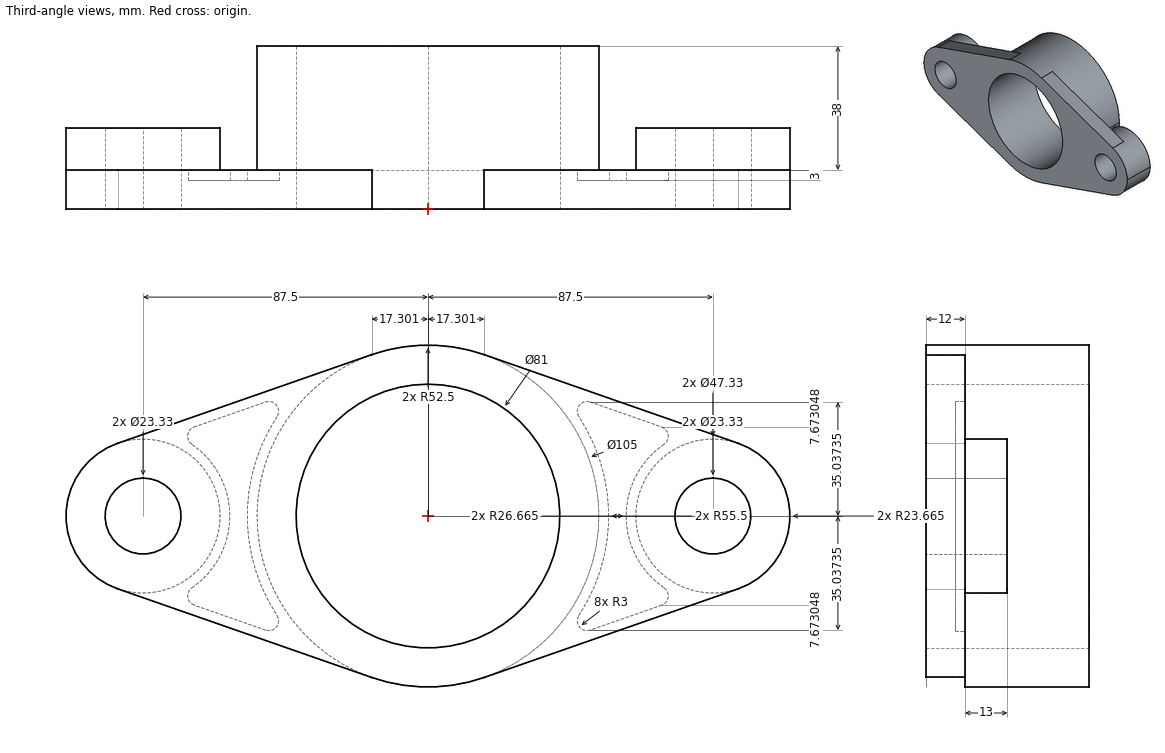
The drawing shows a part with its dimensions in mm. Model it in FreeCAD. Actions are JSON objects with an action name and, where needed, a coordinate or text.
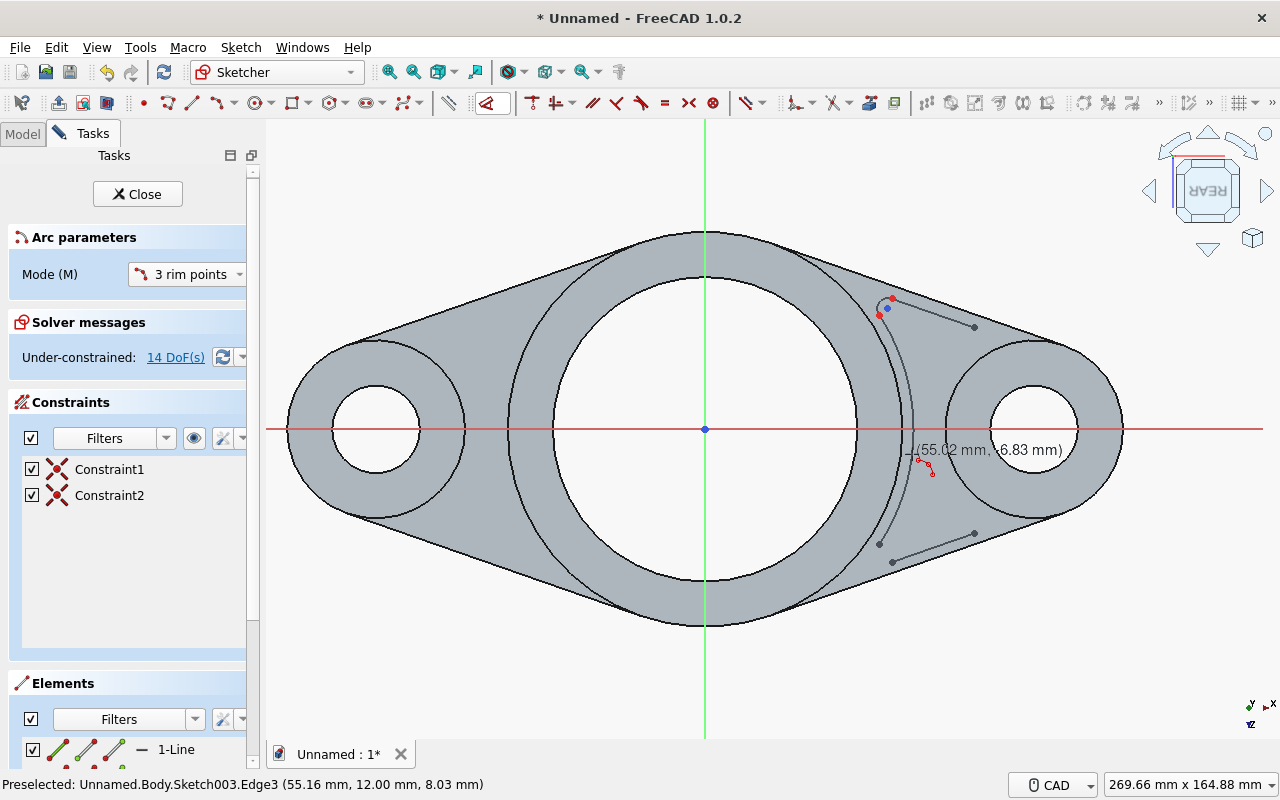
{"action": "left_click", "coordinate": [879, 545]}
{"action": "left_click", "coordinate": [892, 562]}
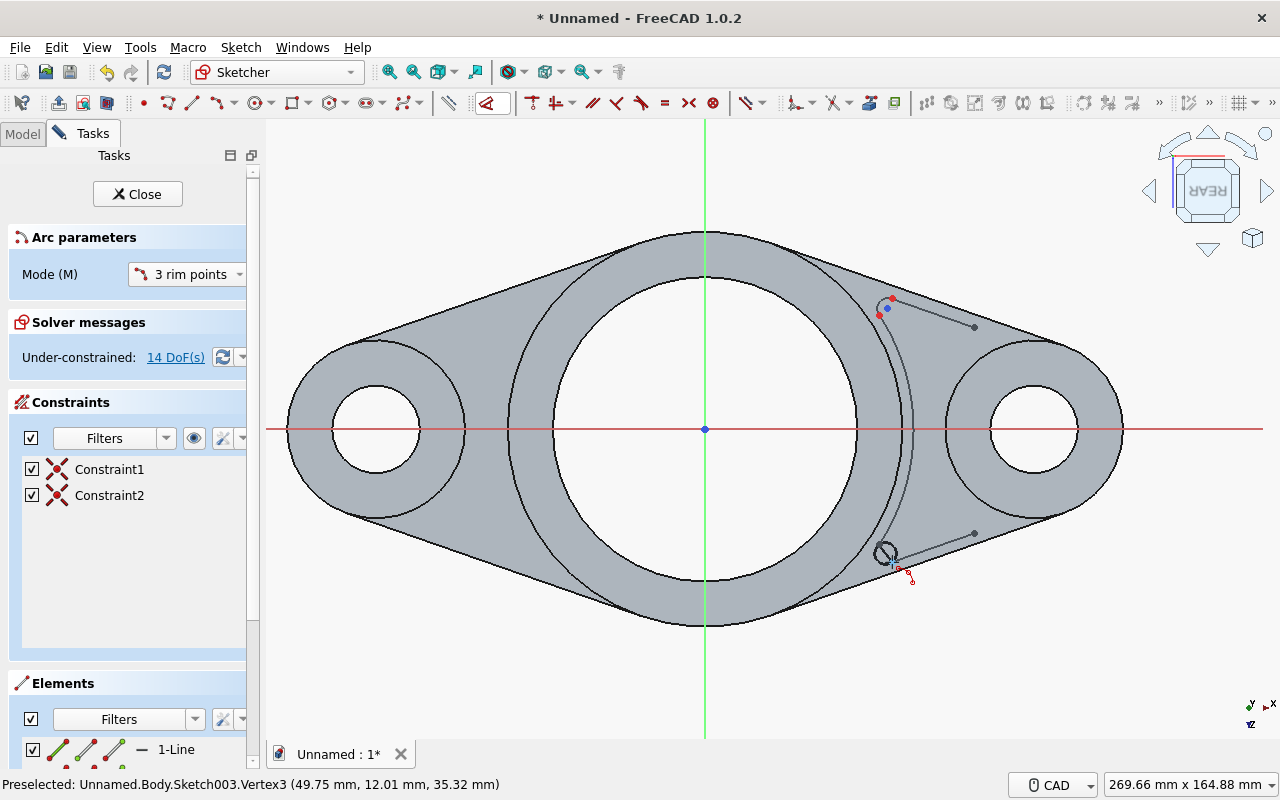
{"action": "scroll", "coordinate": [880, 557], "scroll_direction": "up", "scroll_amount": 4}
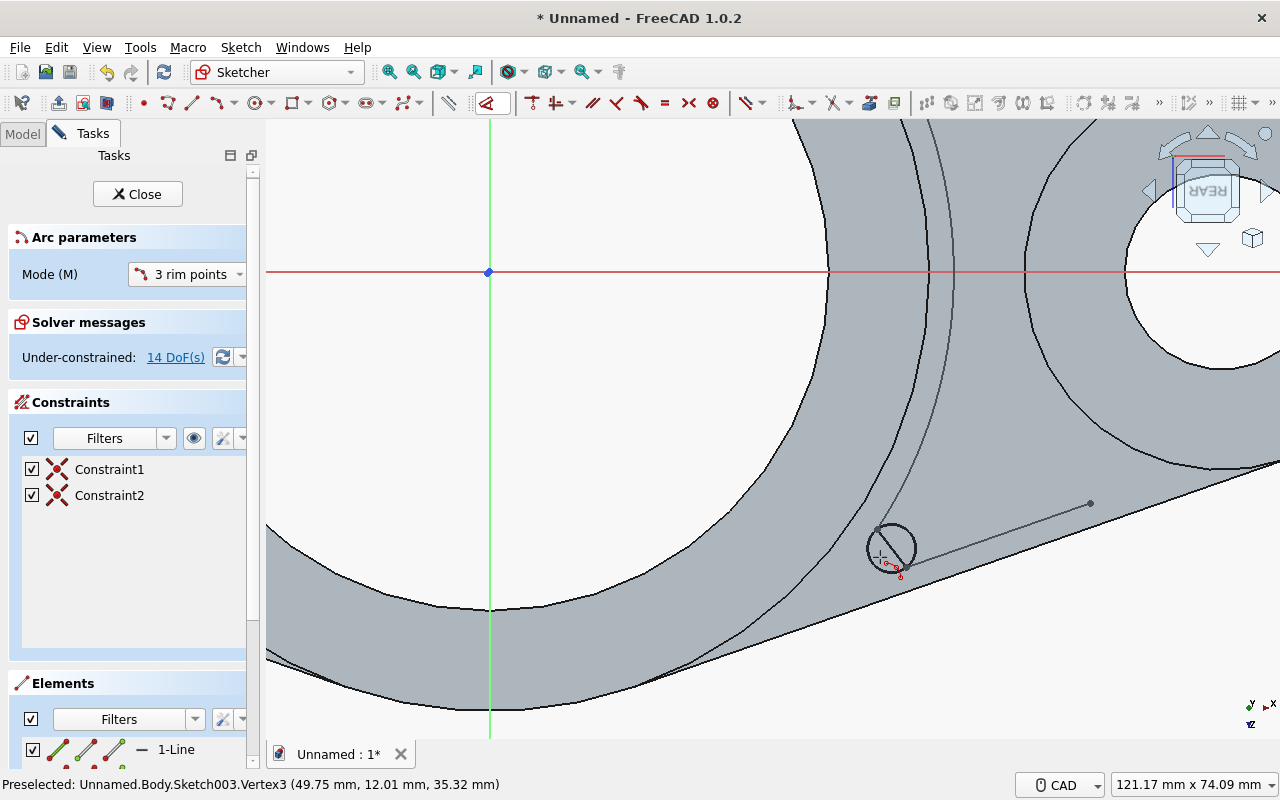
{"action": "left_click", "coordinate": [879, 557]}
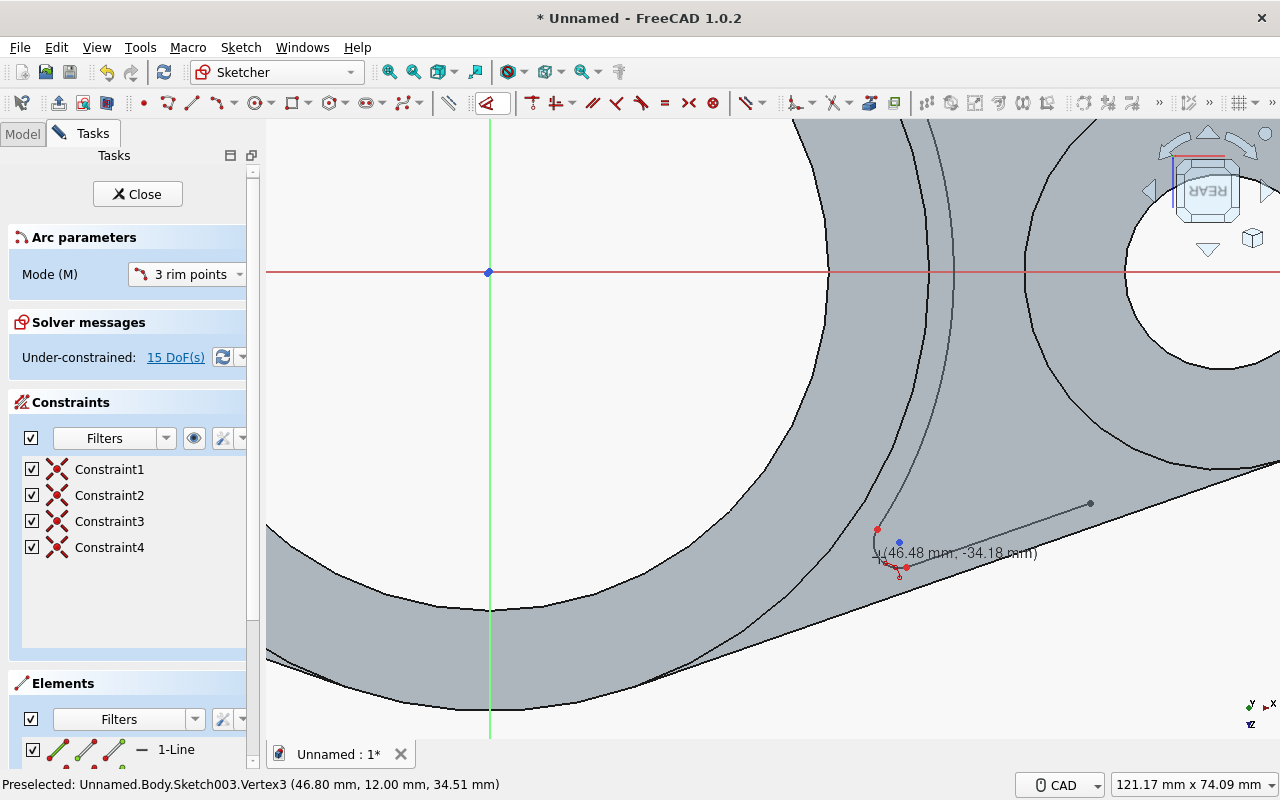
{"action": "left_click", "coordinate": [1090, 503]}
{"action": "left_click", "coordinate": [1097, 456]}
{"action": "left_click", "coordinate": [1108, 481]}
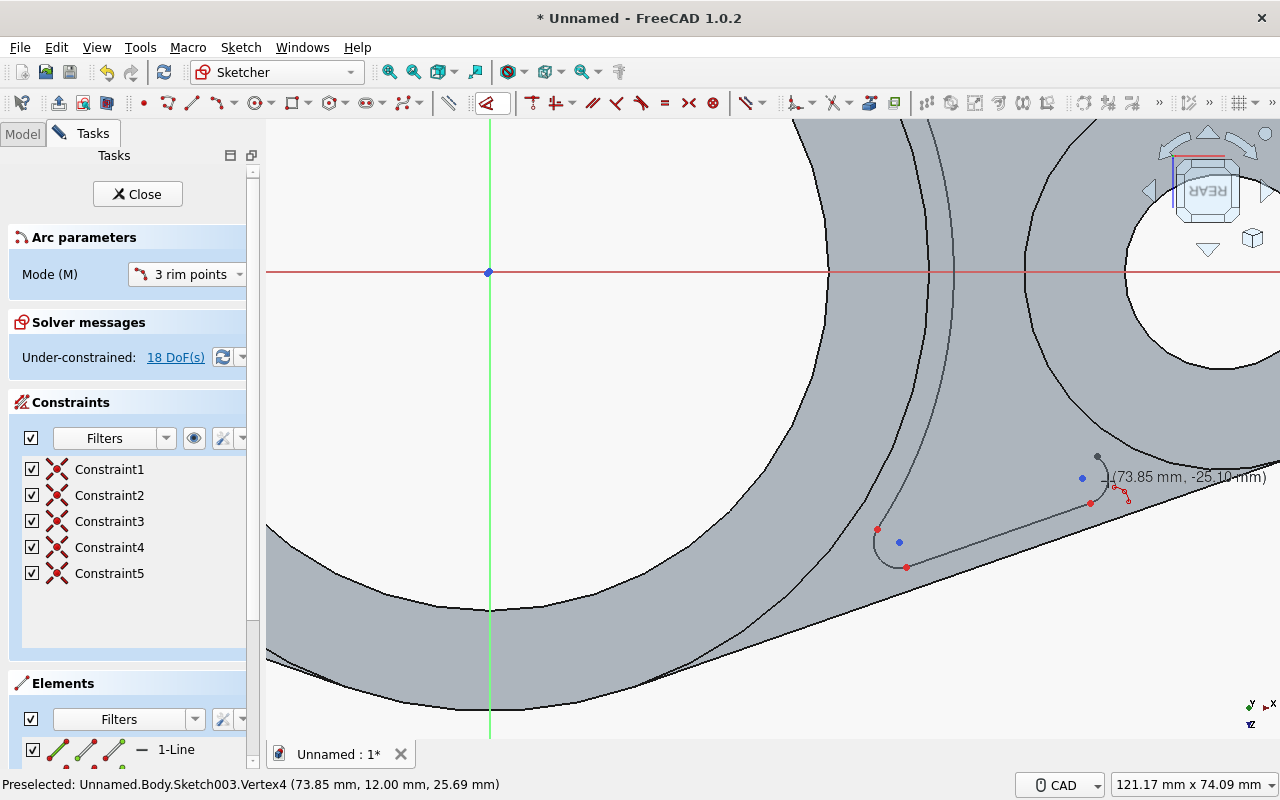
{"action": "left_click", "coordinate": [1097, 457]}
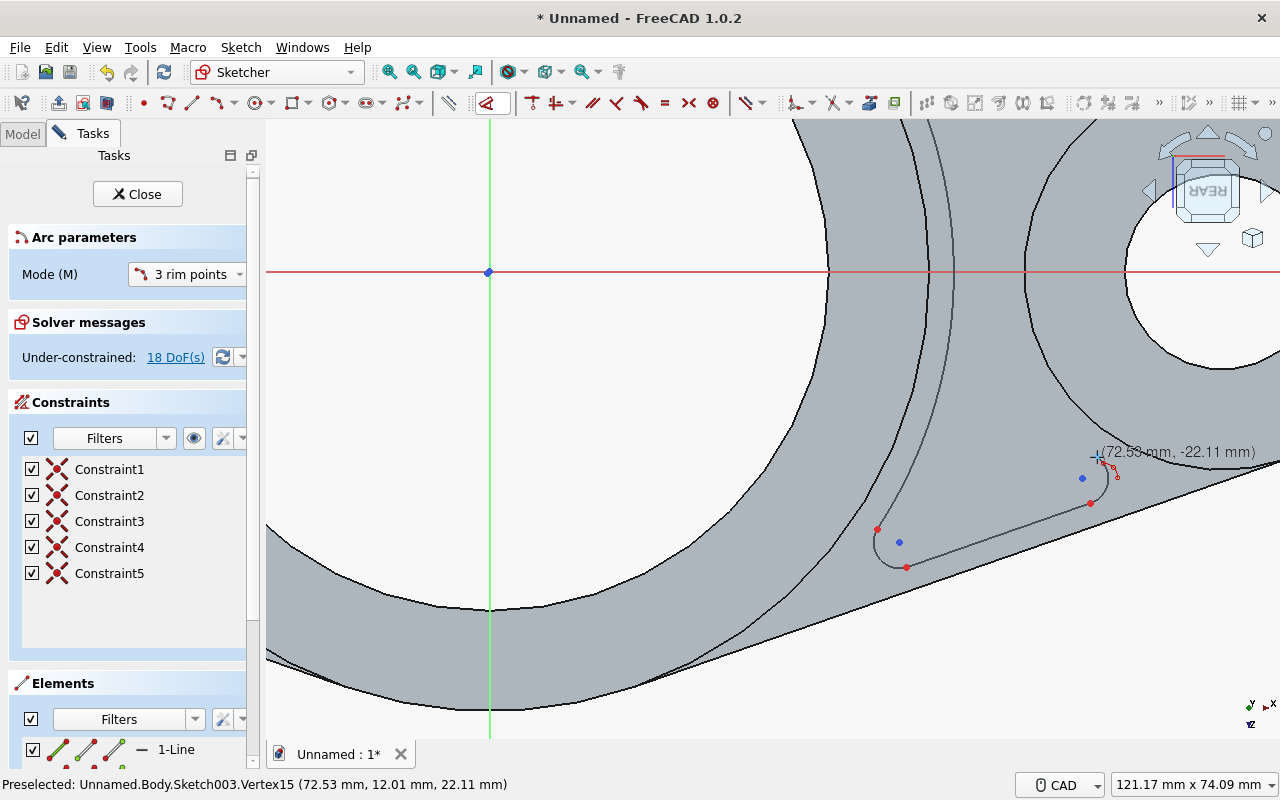
{"action": "scroll", "coordinate": [880, 557], "scroll_direction": "down", "scroll_amount": 4}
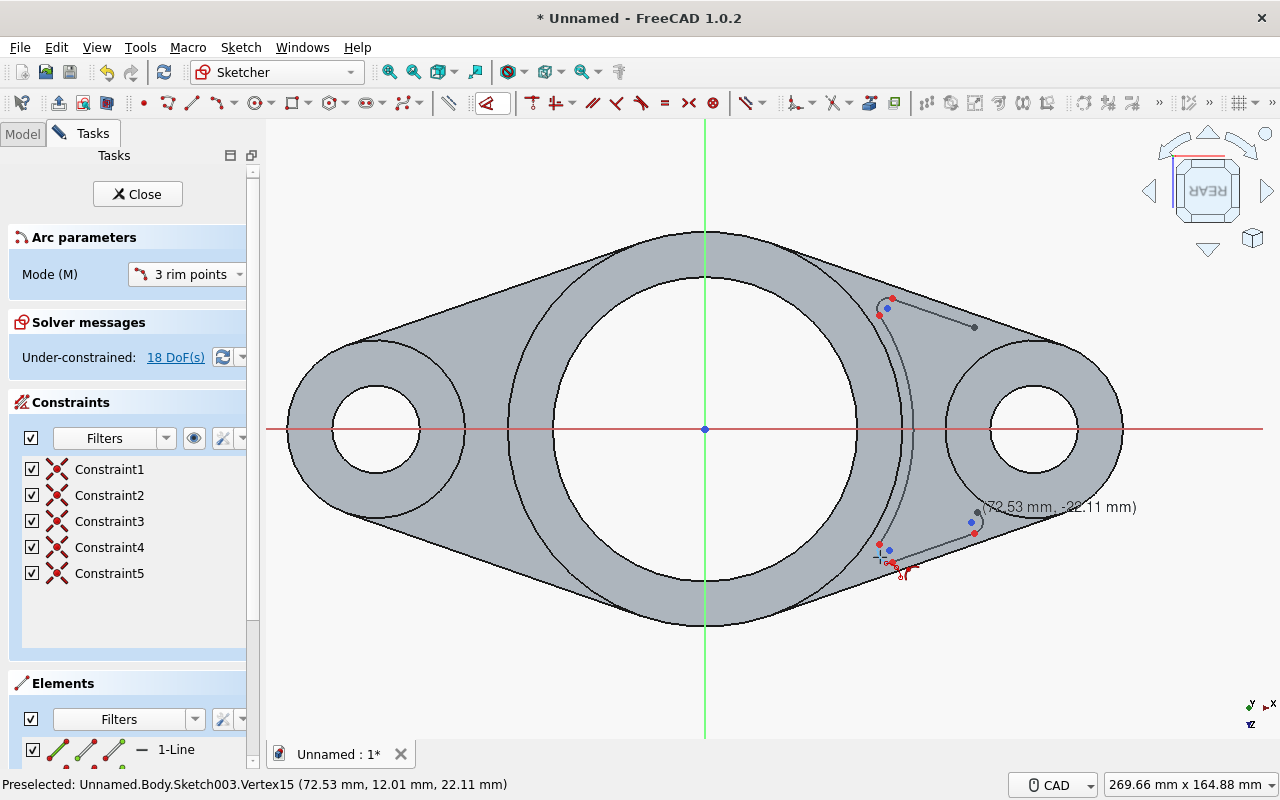
{"action": "left_click", "coordinate": [978, 346]}
{"action": "left_click", "coordinate": [936, 410]}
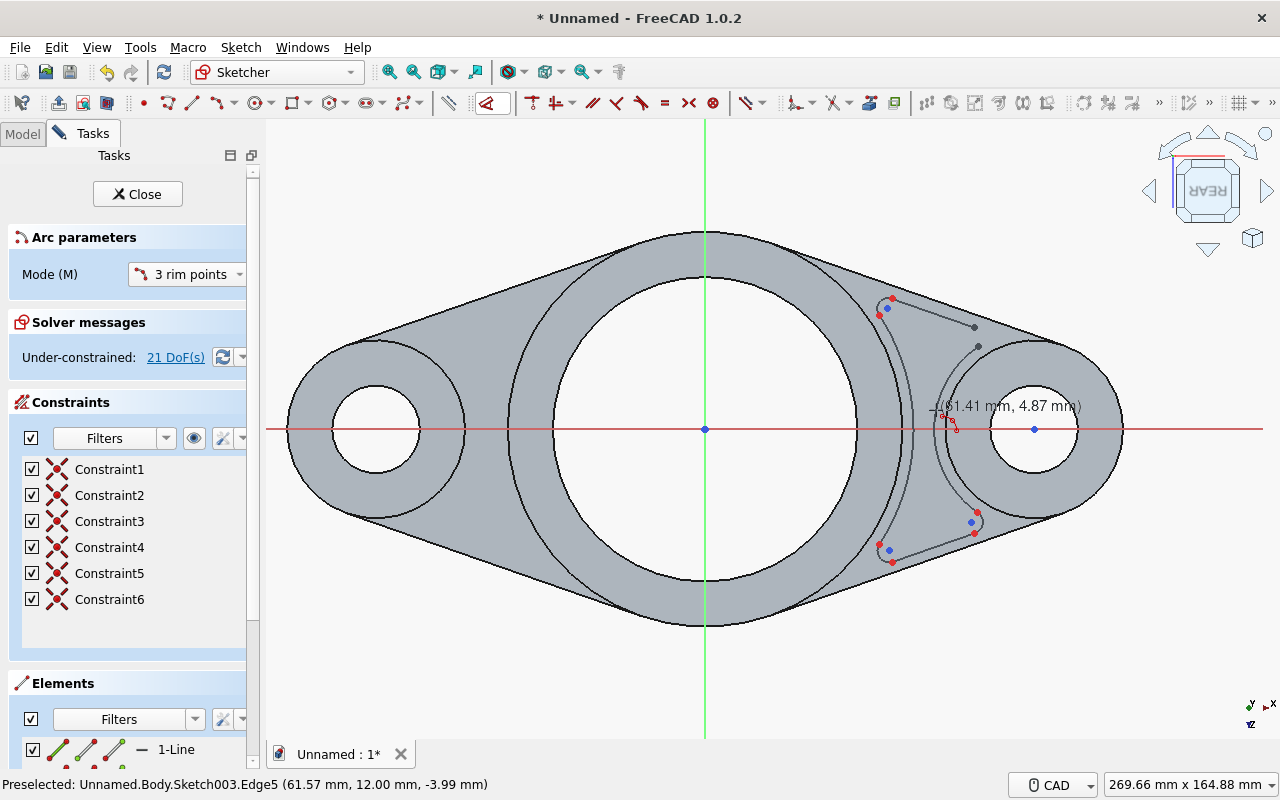
{"action": "left_click", "coordinate": [978, 347]}
{"action": "left_click", "coordinate": [975, 328]}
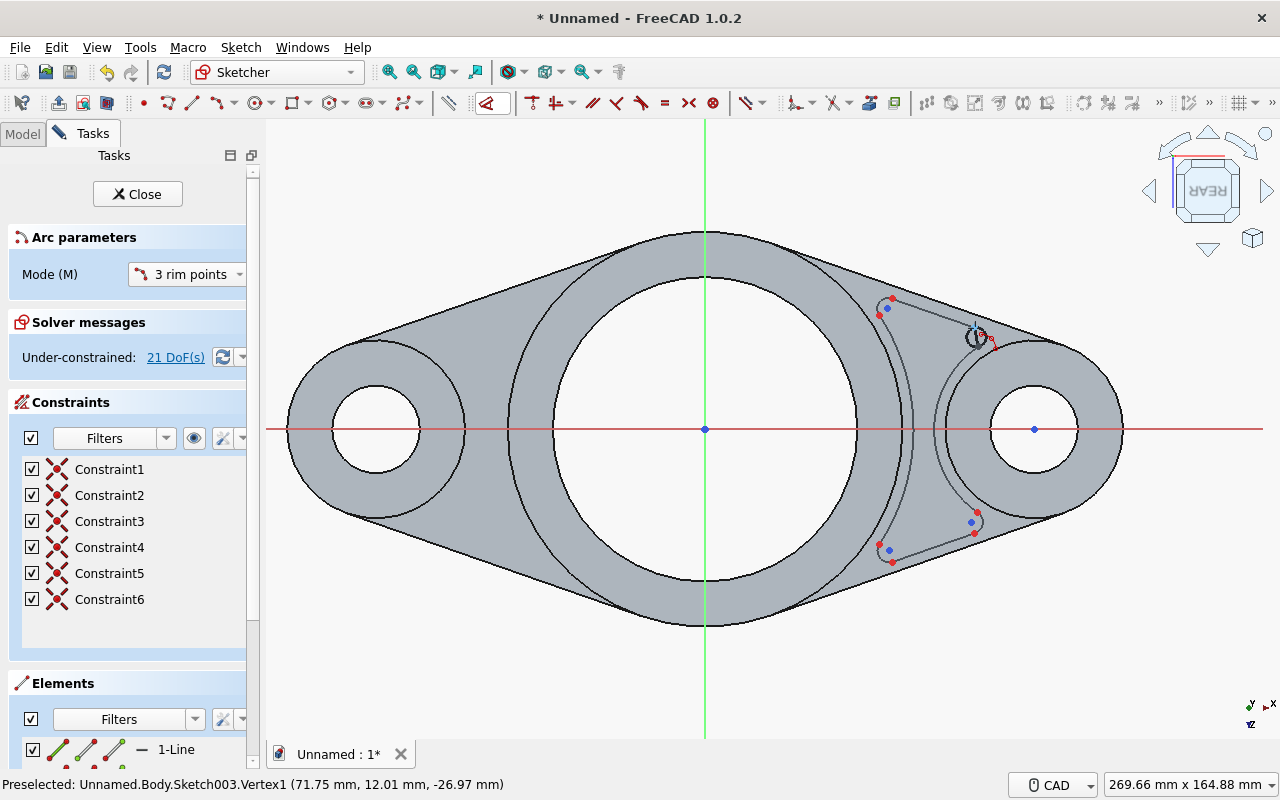
{"action": "scroll", "coordinate": [983, 336], "scroll_direction": "up", "scroll_amount": 5}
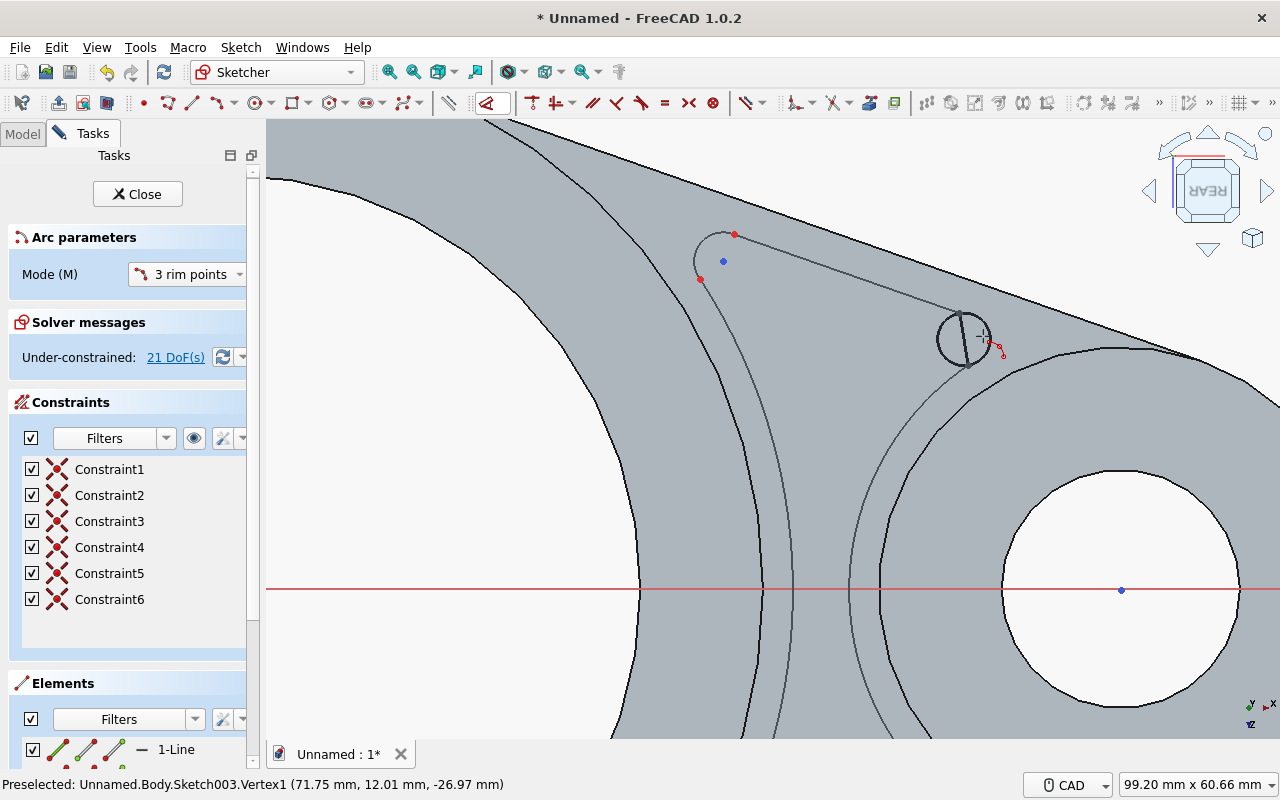
{"action": "left_click", "coordinate": [981, 334]}